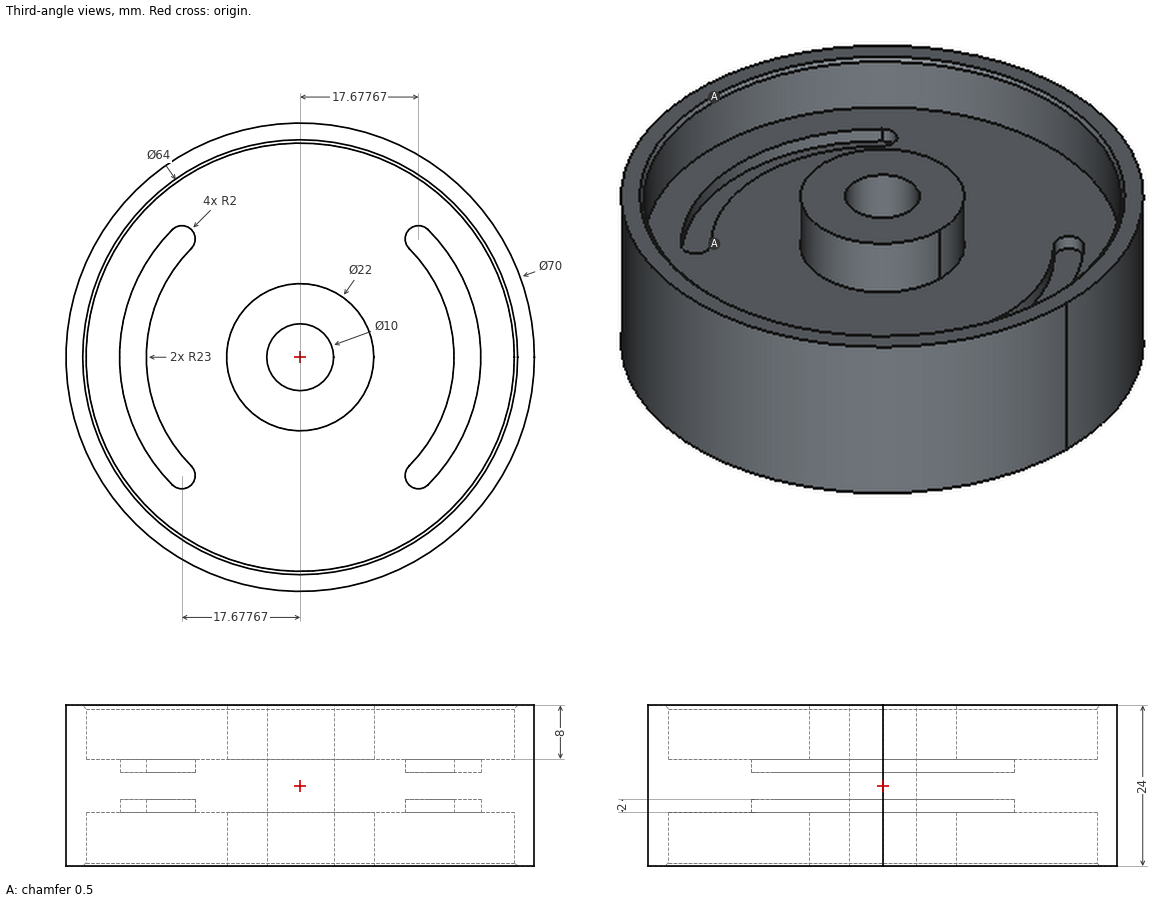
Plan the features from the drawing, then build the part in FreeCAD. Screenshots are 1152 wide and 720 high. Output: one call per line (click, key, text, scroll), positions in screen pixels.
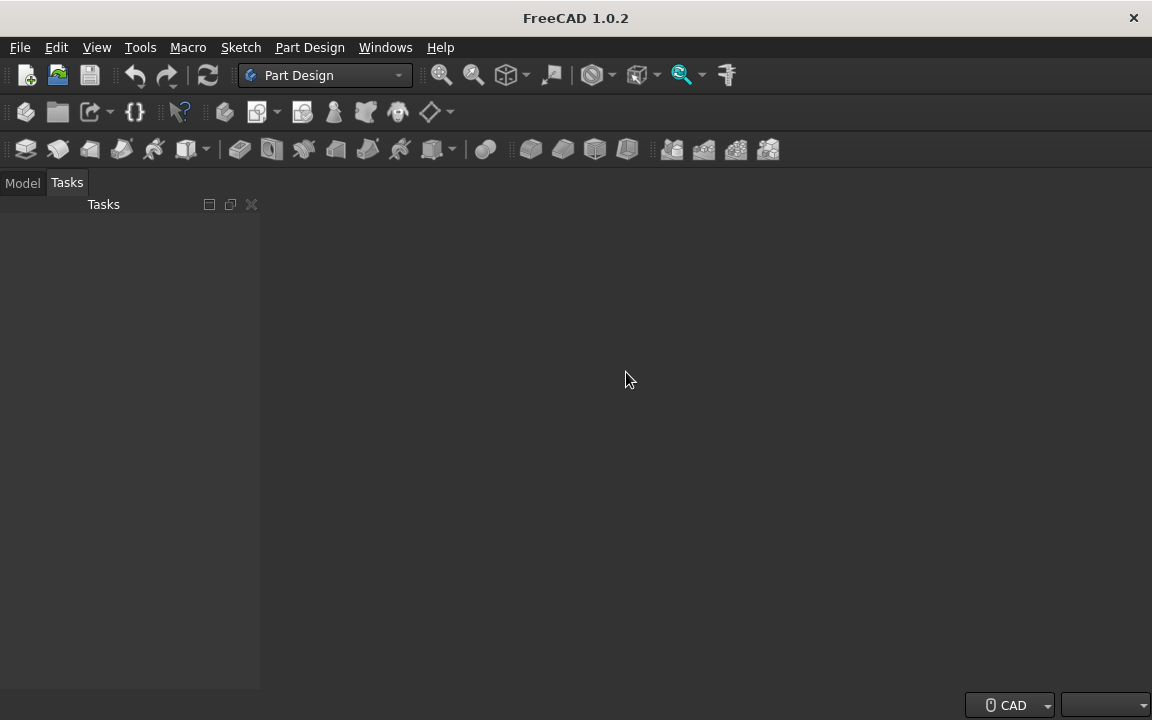
key(ctrl+n)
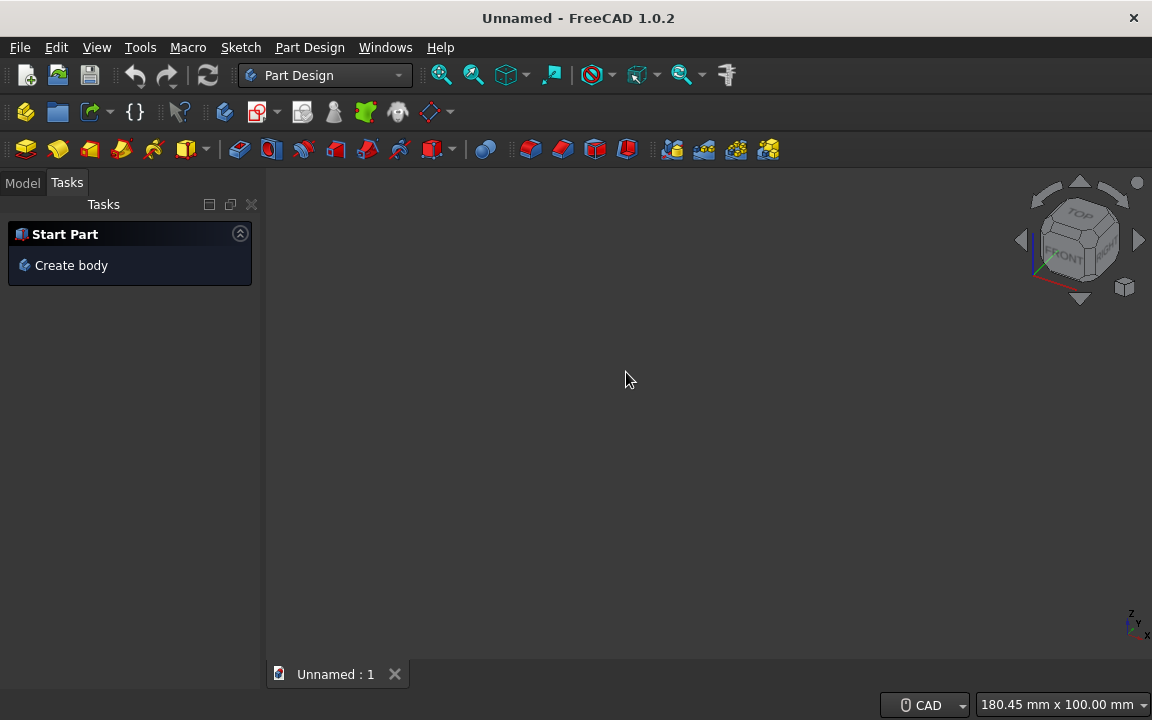
click(258, 112)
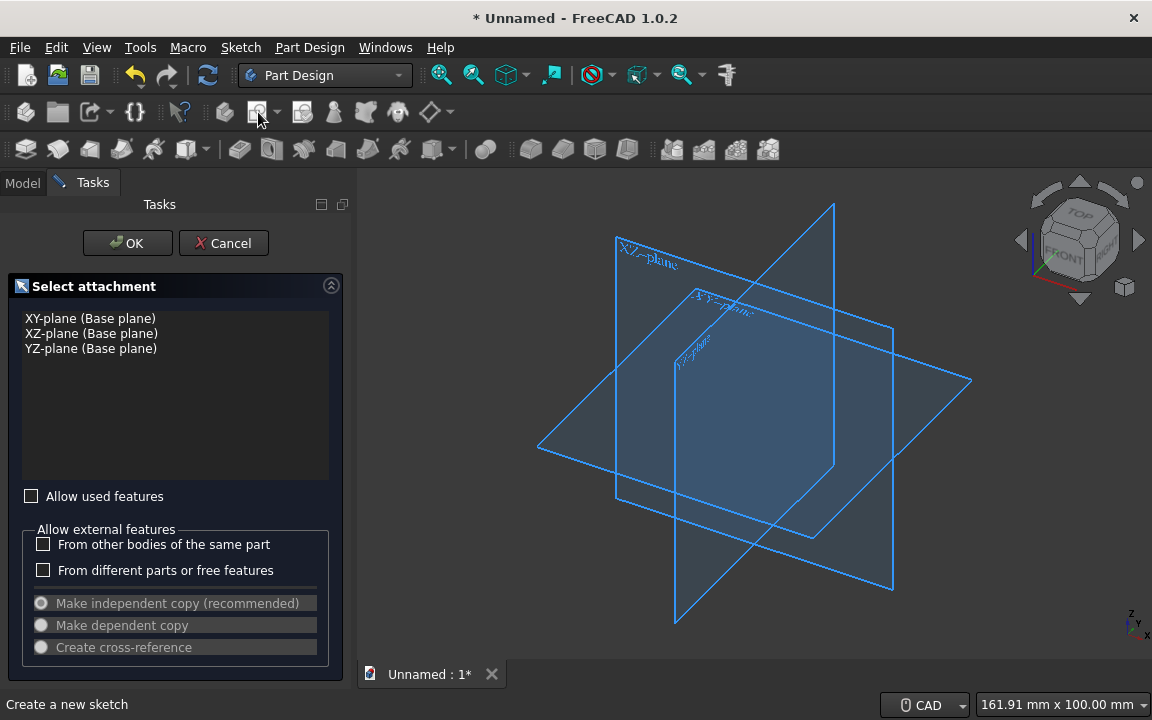
click(82, 318)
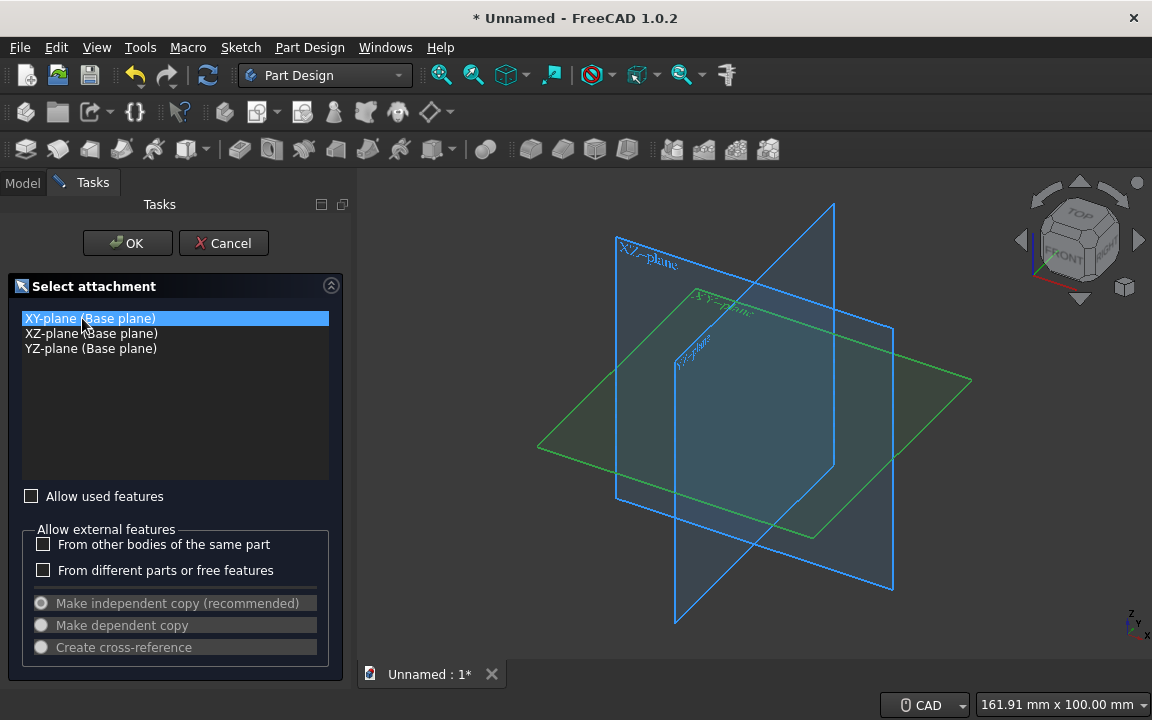
click(128, 243)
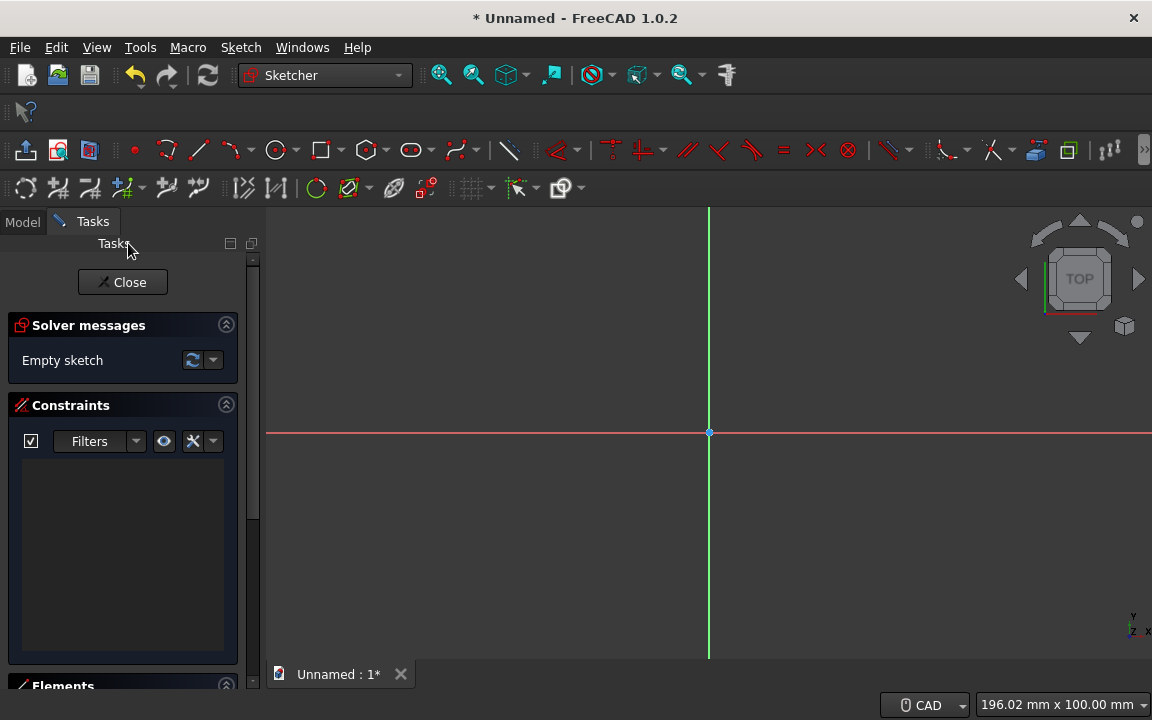
key(g)
key(c)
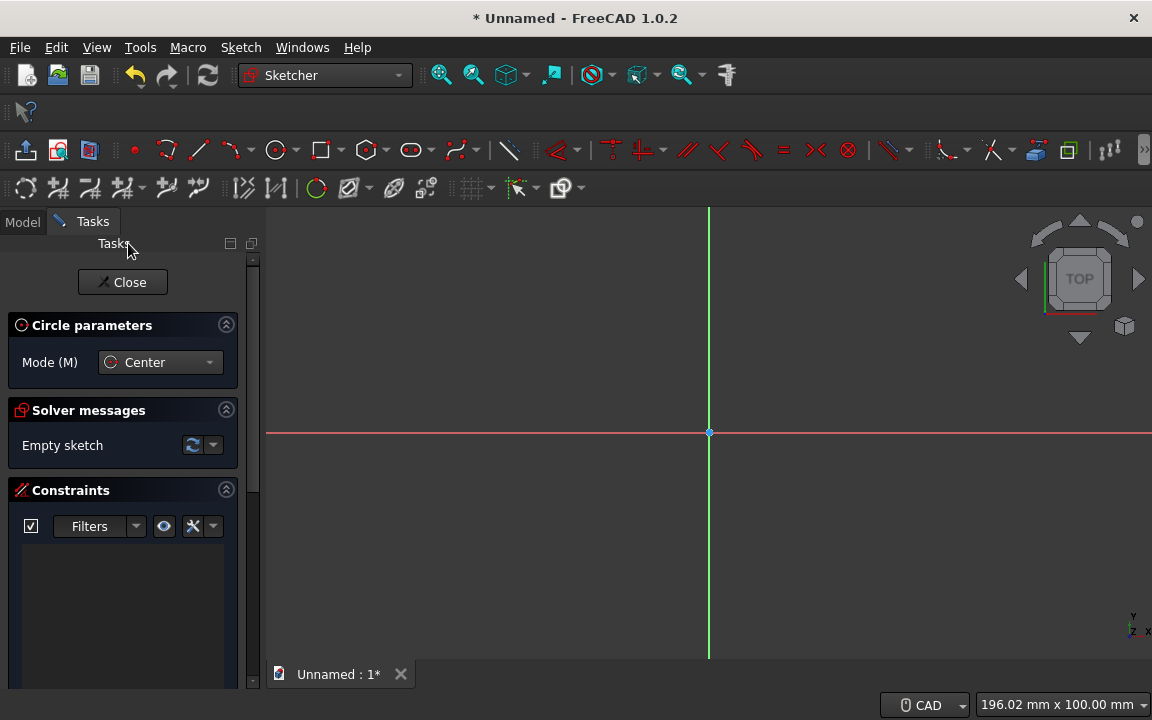
click(709, 433)
move(821, 321)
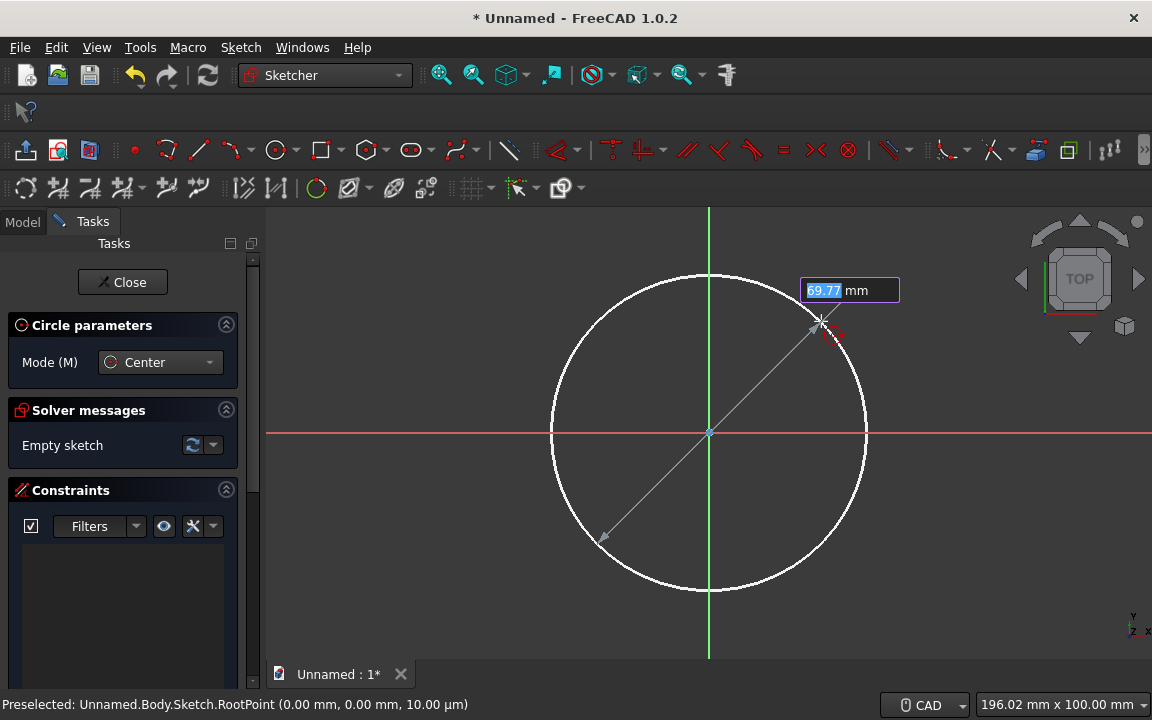
text(70)
key(Return)
key(Escape)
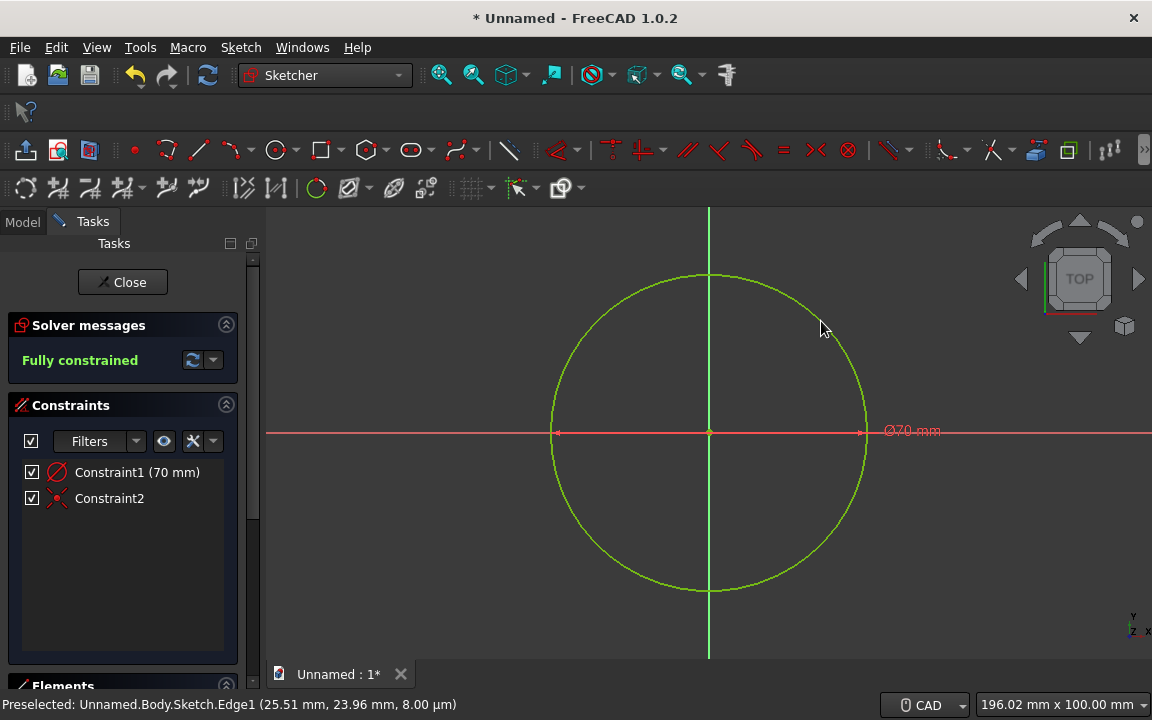
click(123, 282)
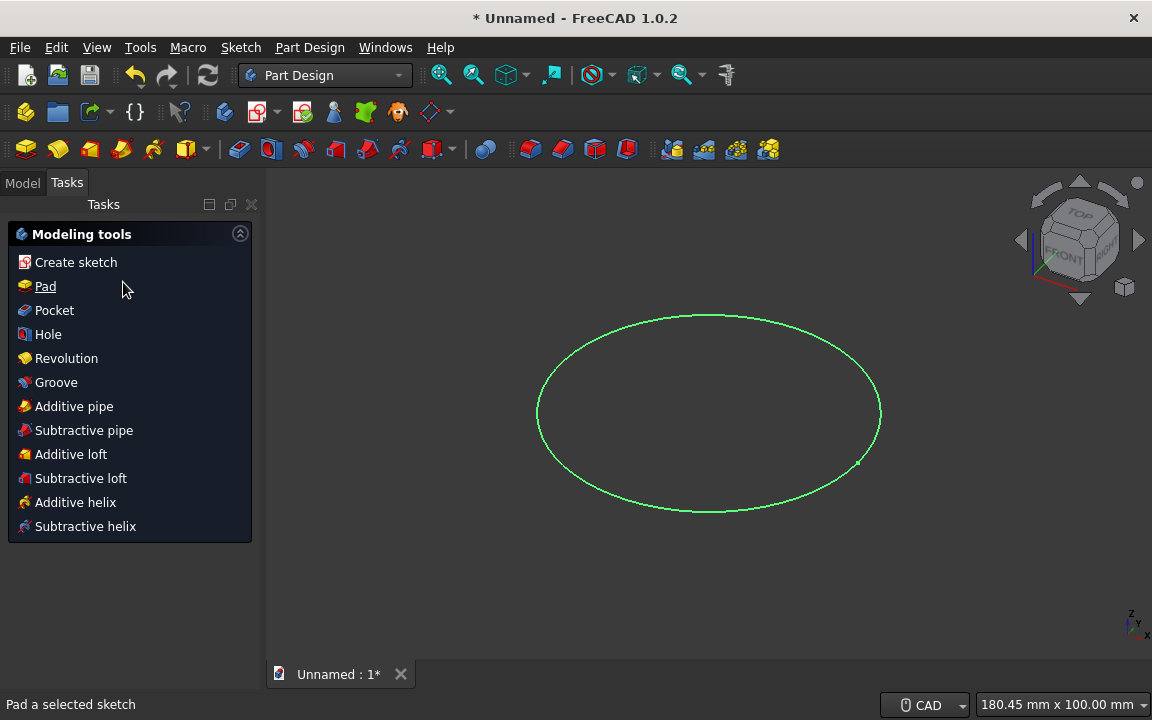
click(26, 150)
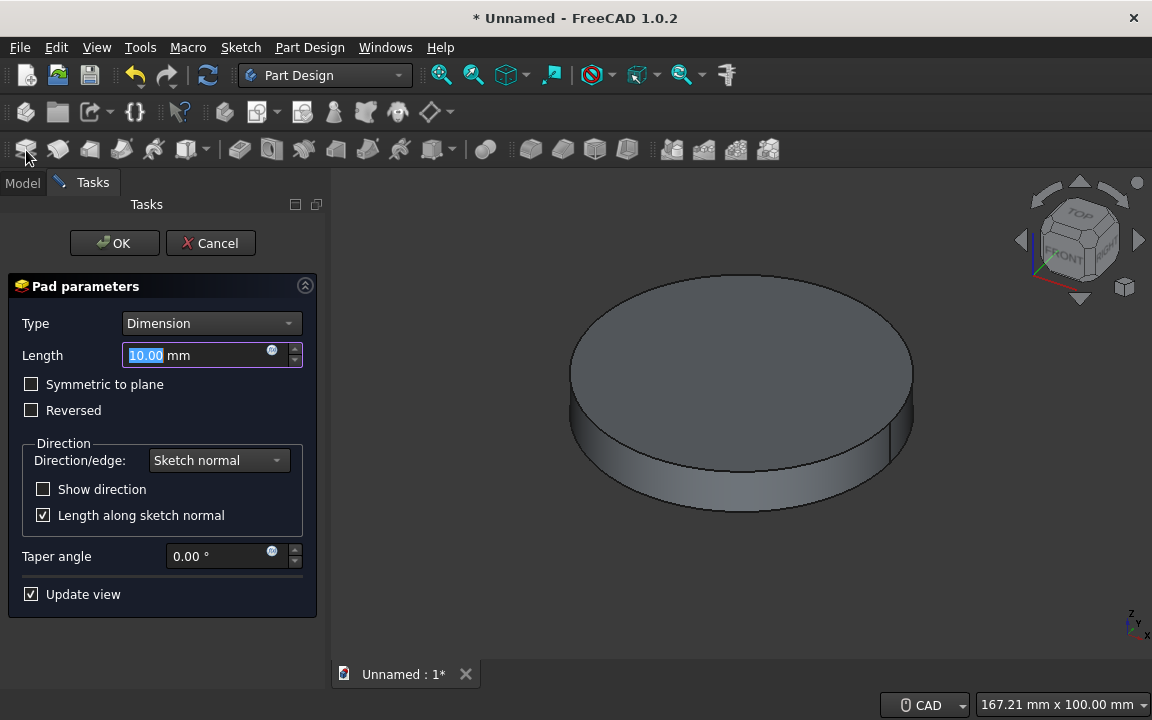
text(24)
key(Tab)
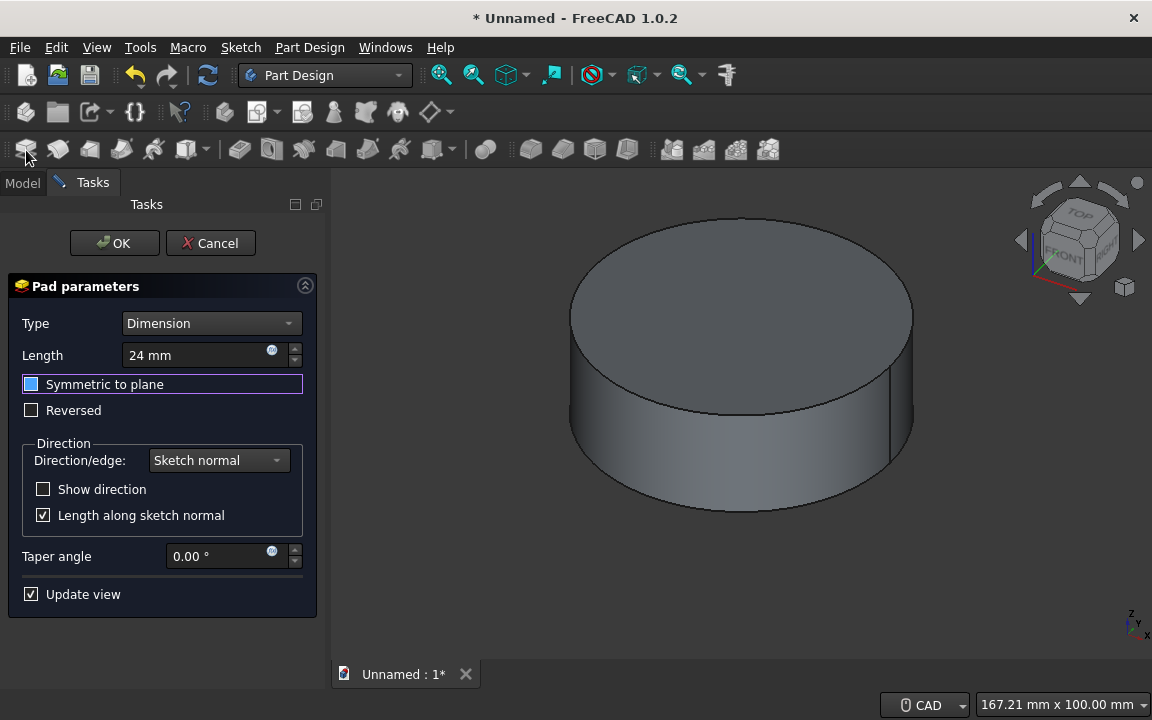
click(30, 384)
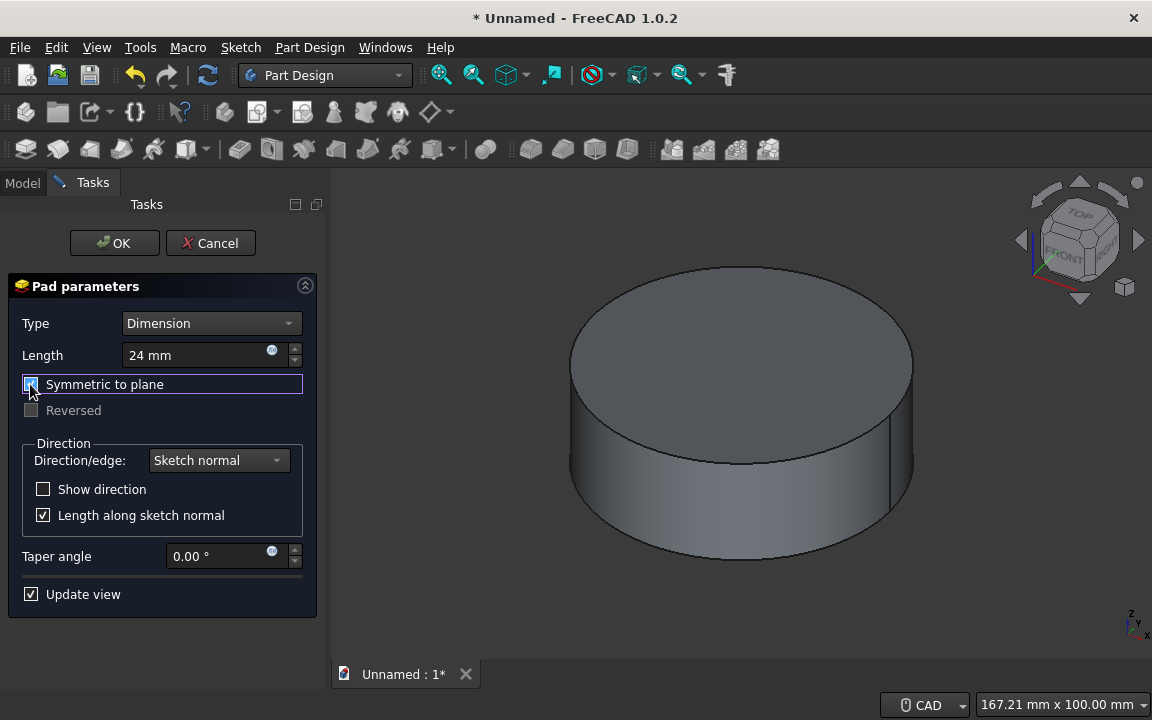
click(115, 243)